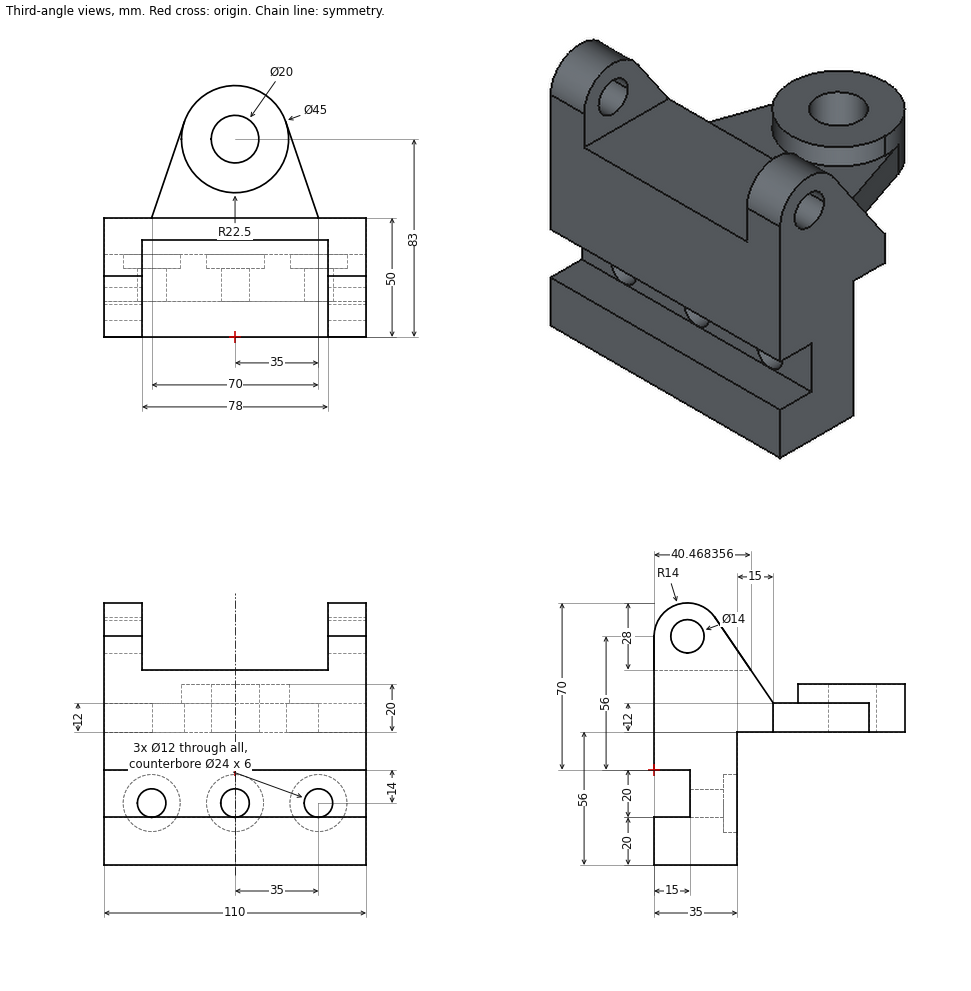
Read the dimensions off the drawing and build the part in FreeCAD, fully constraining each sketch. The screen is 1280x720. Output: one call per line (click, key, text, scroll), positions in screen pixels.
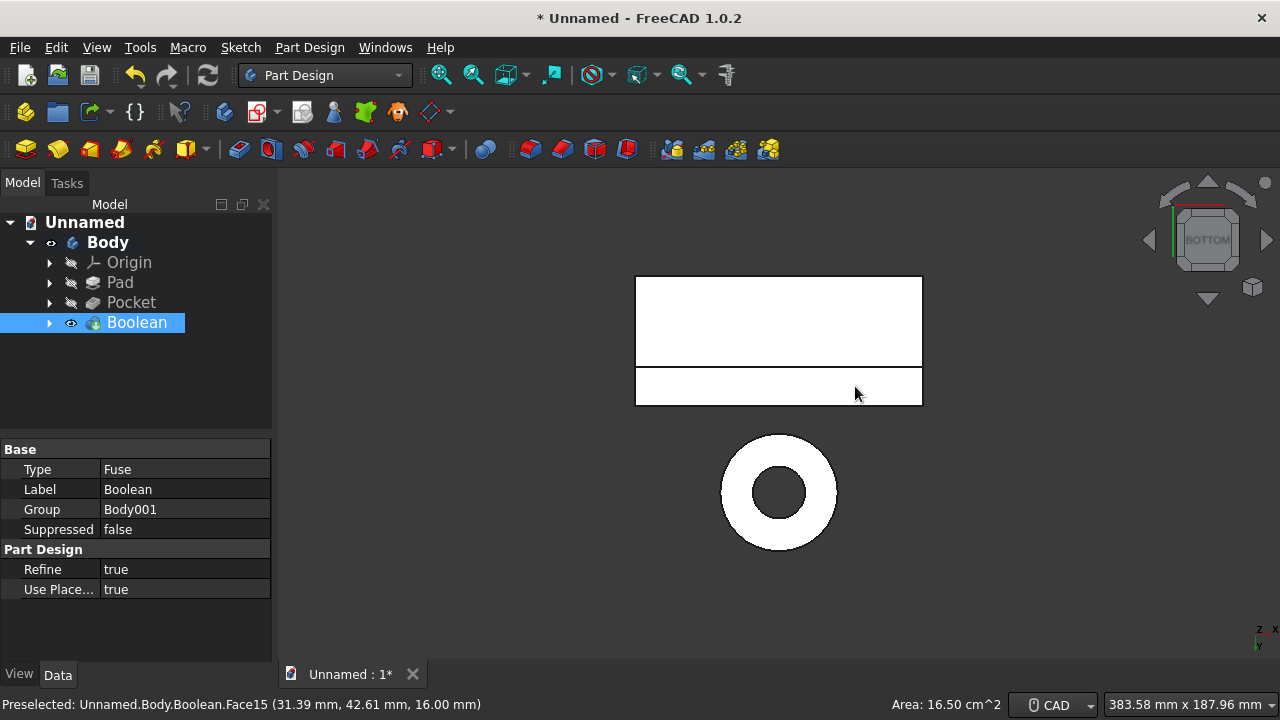
click(258, 112)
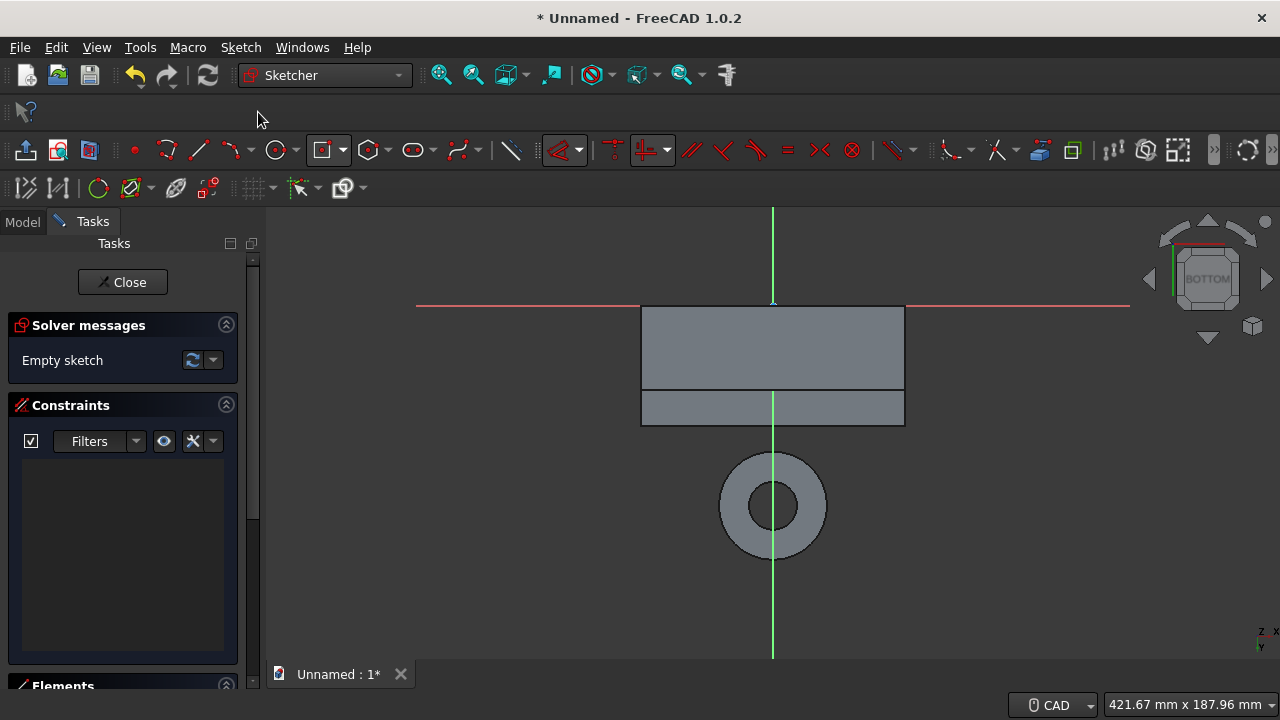
click(90, 150)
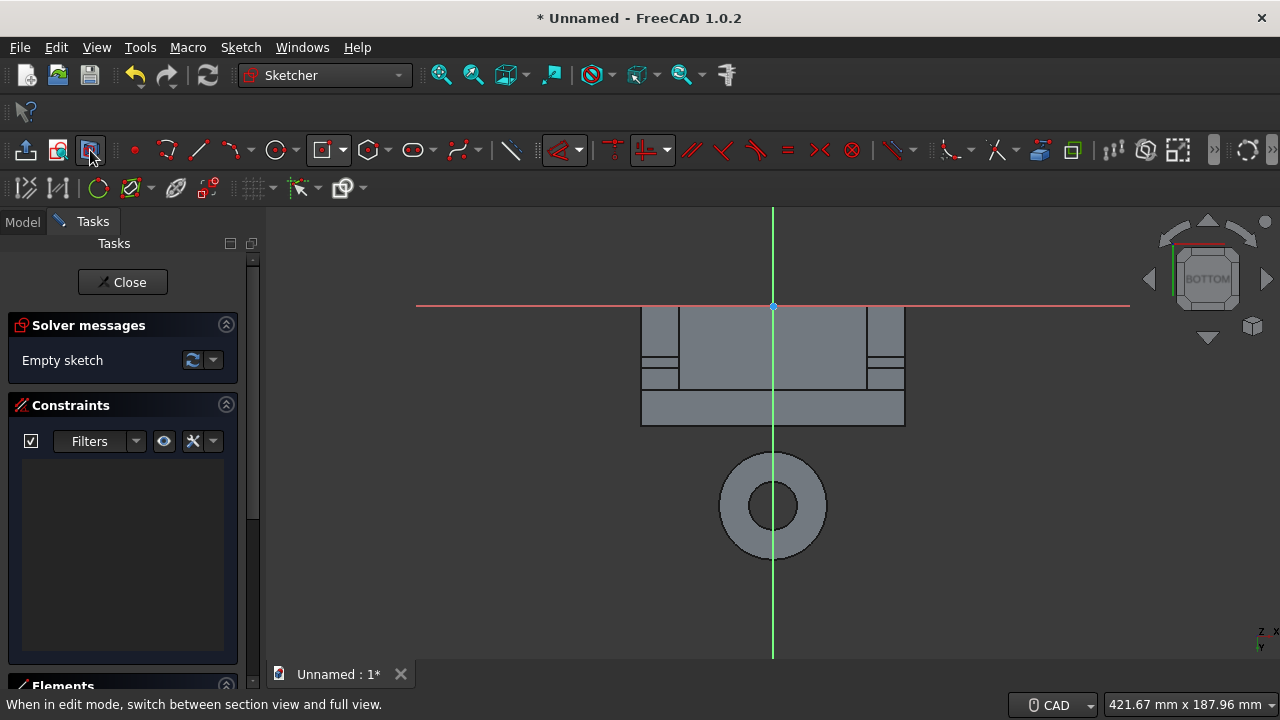
key(g)
key(m)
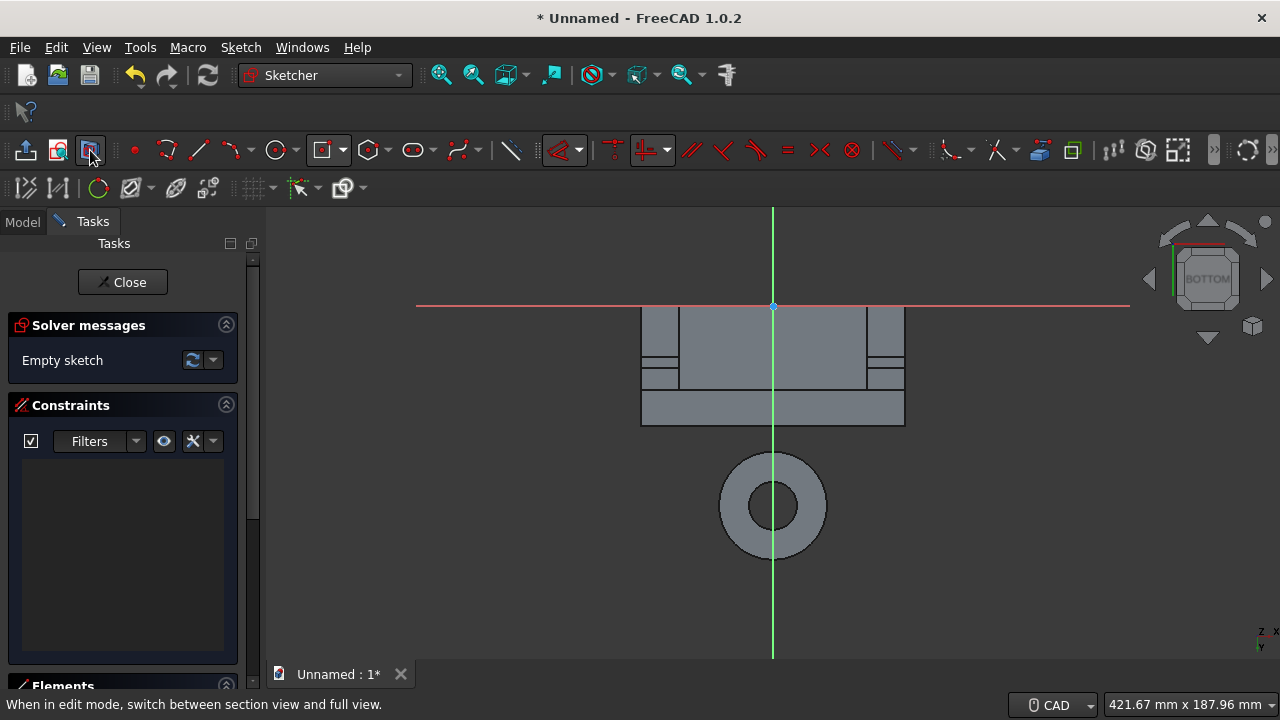
click(824, 523)
click(857, 426)
click(689, 426)
click(722, 523)
right_click(722, 523)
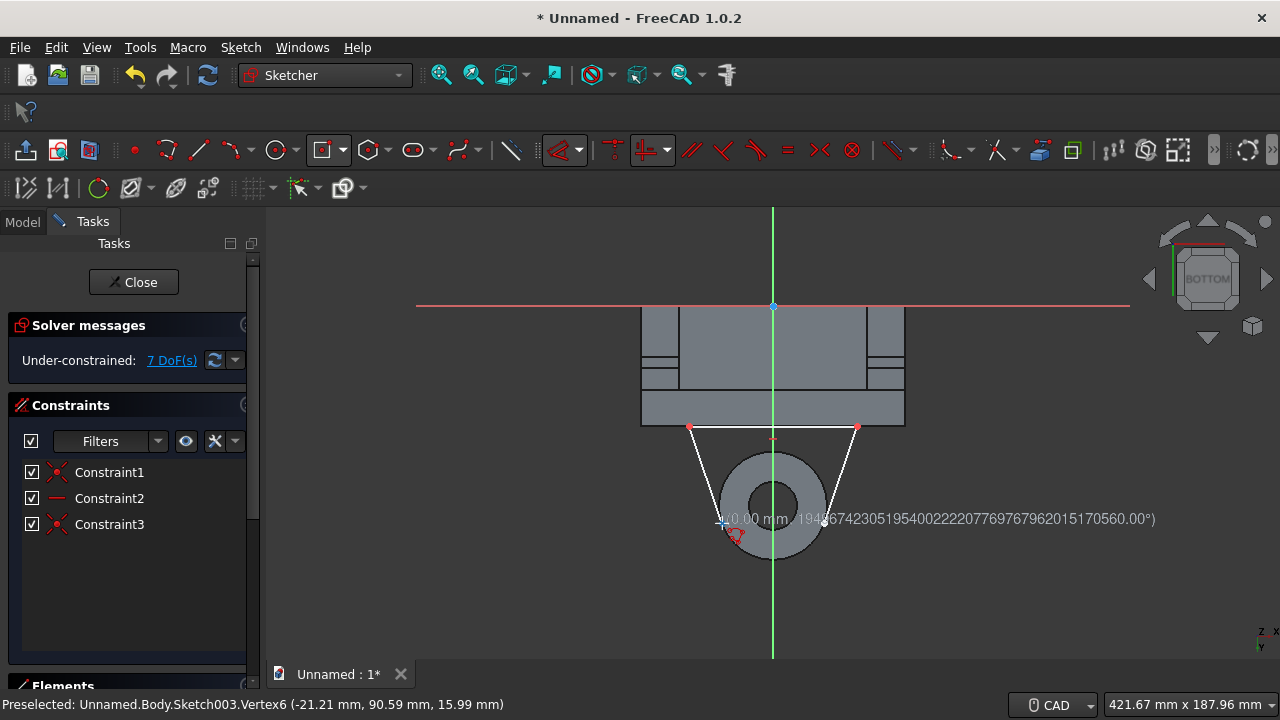
click(232, 150)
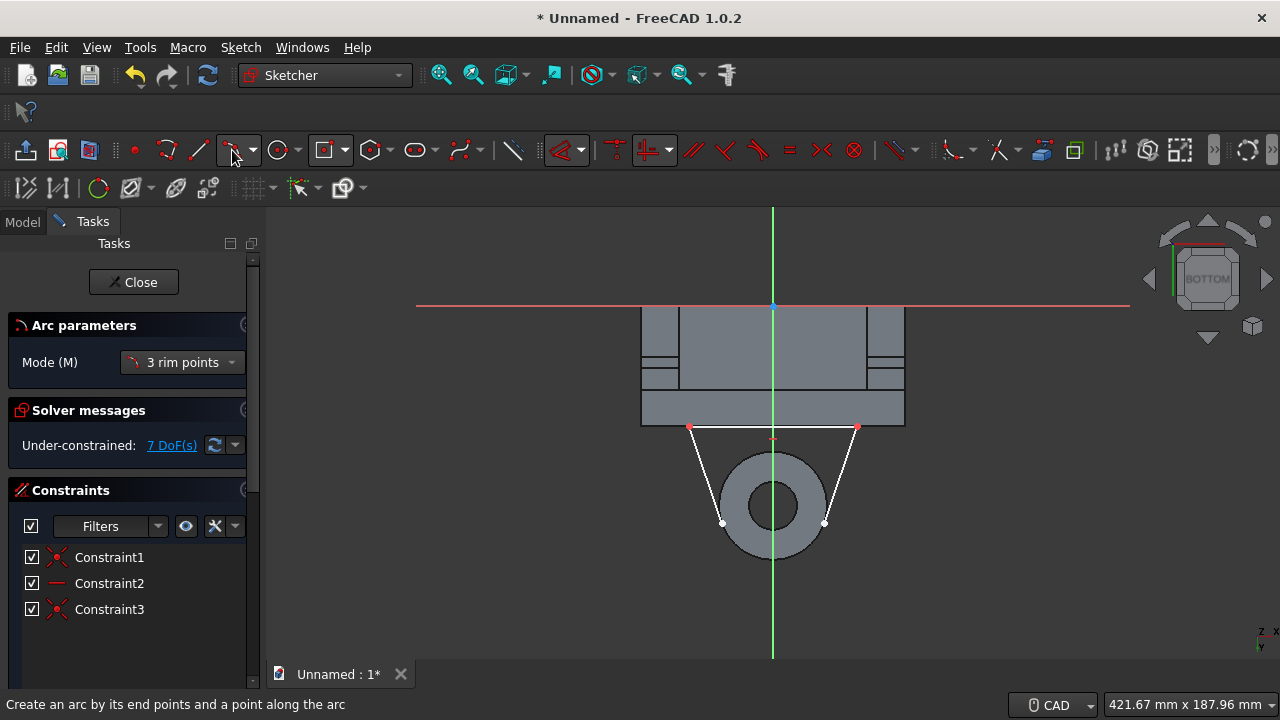
click(722, 524)
click(824, 524)
click(793, 455)
key(Escape)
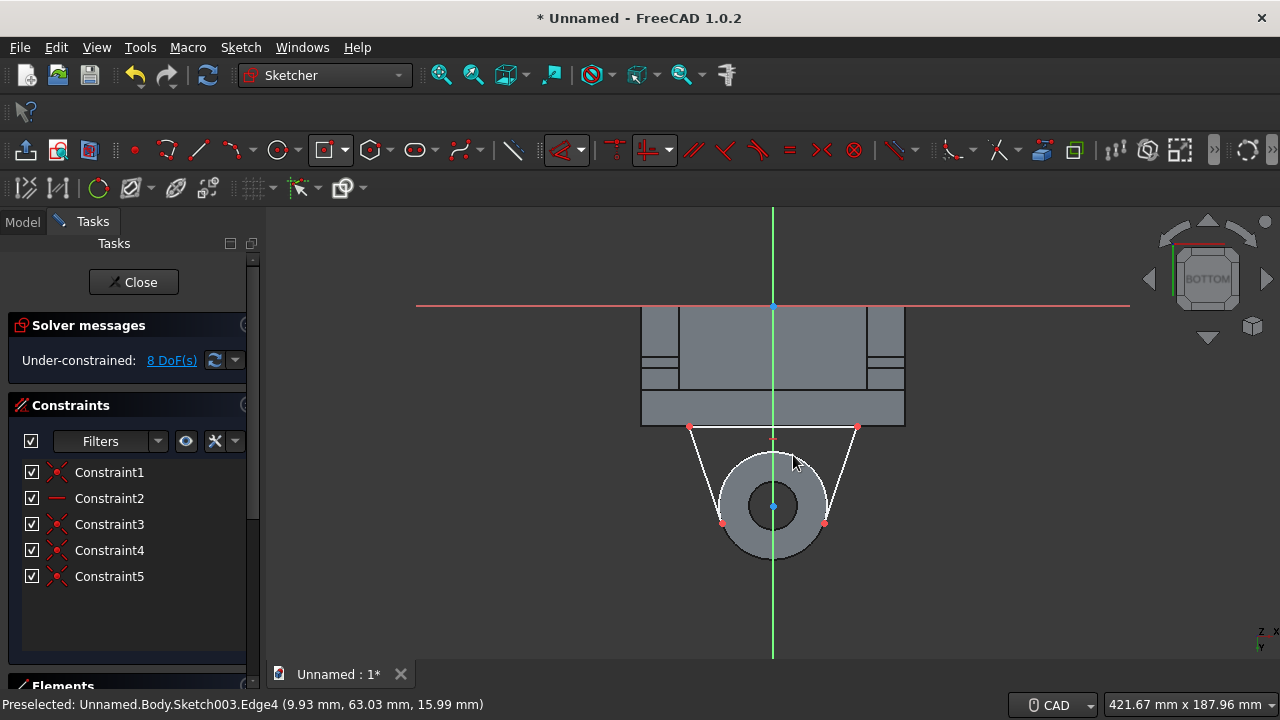
click(847, 456)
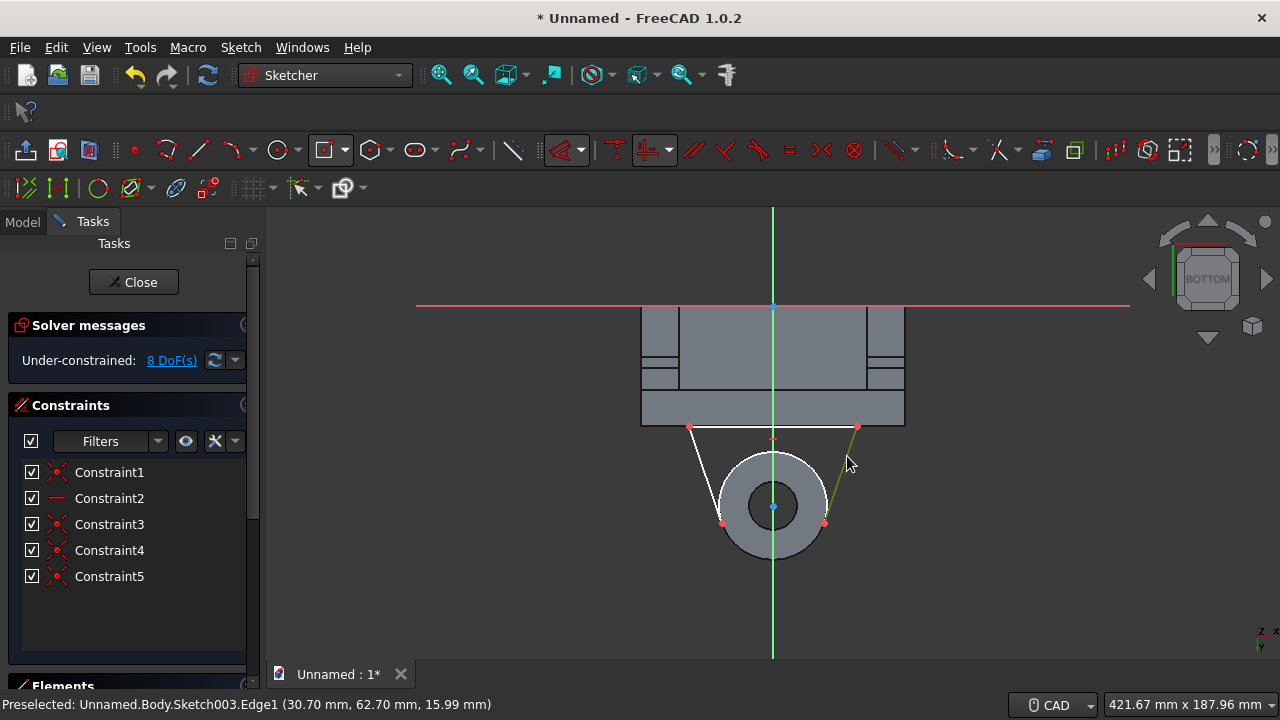
click(810, 467)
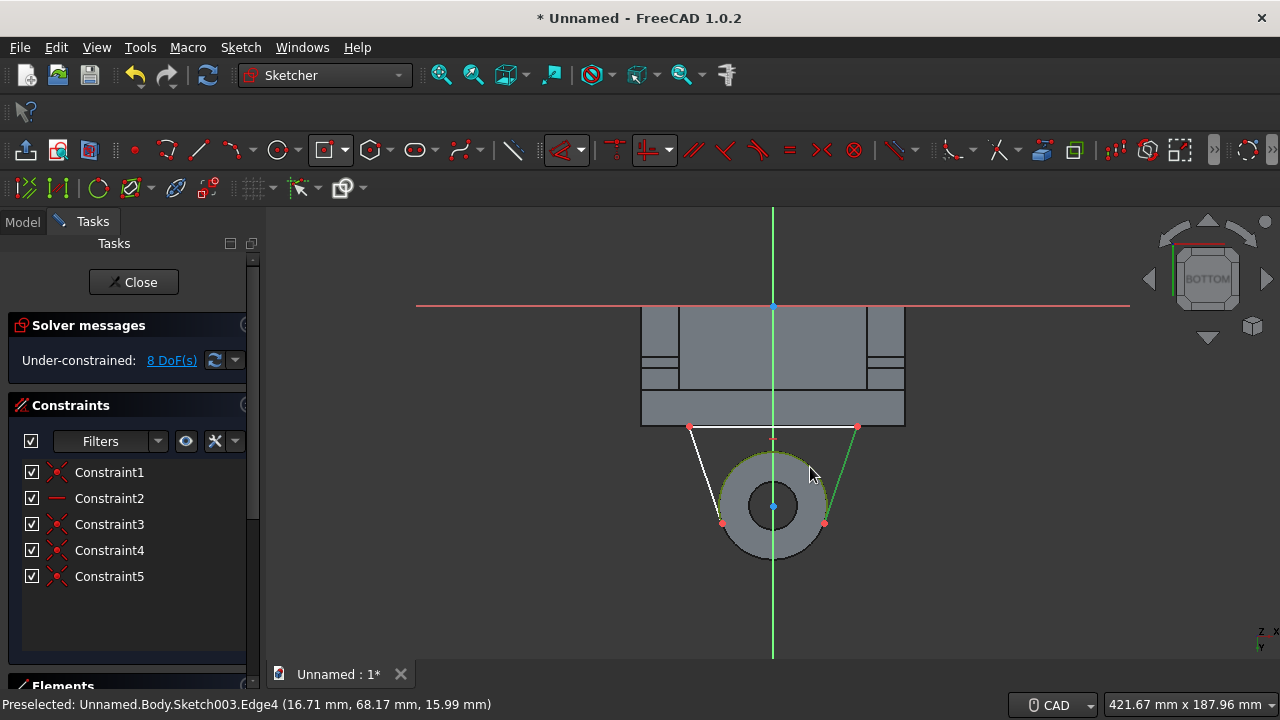
click(758, 150)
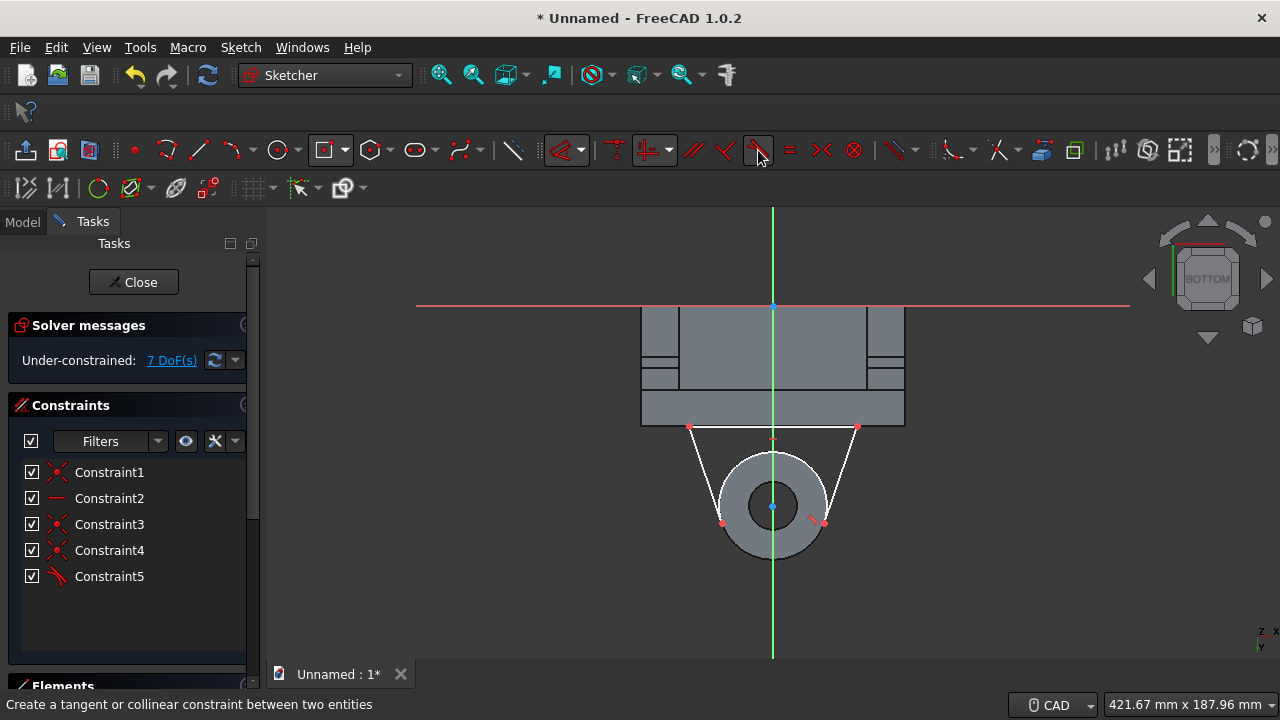
click(699, 456)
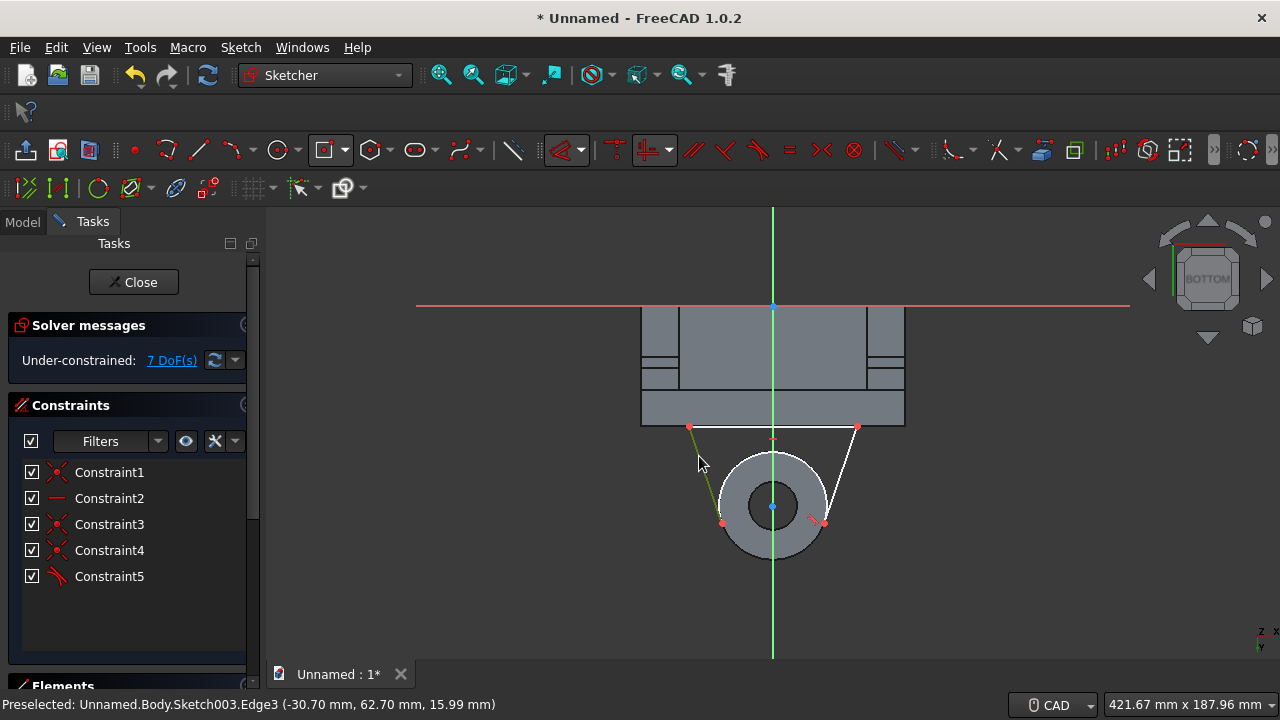
click(810, 467)